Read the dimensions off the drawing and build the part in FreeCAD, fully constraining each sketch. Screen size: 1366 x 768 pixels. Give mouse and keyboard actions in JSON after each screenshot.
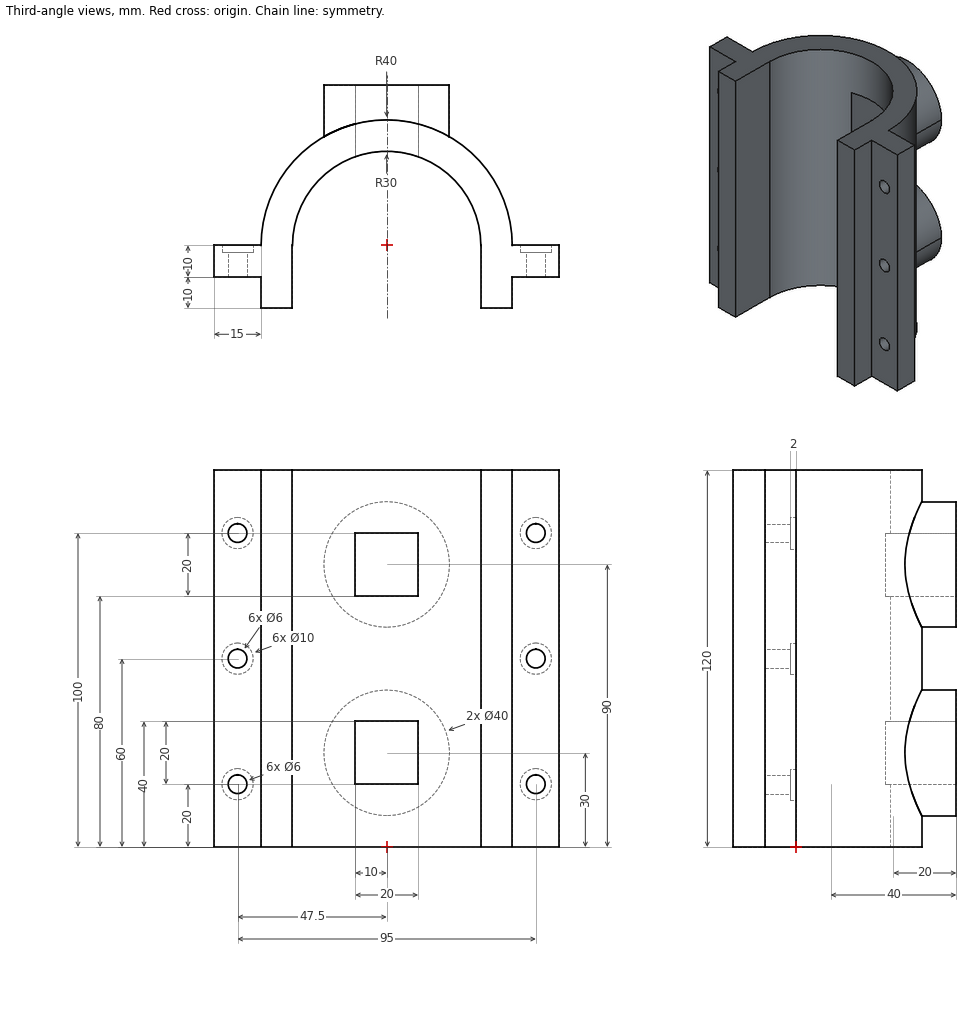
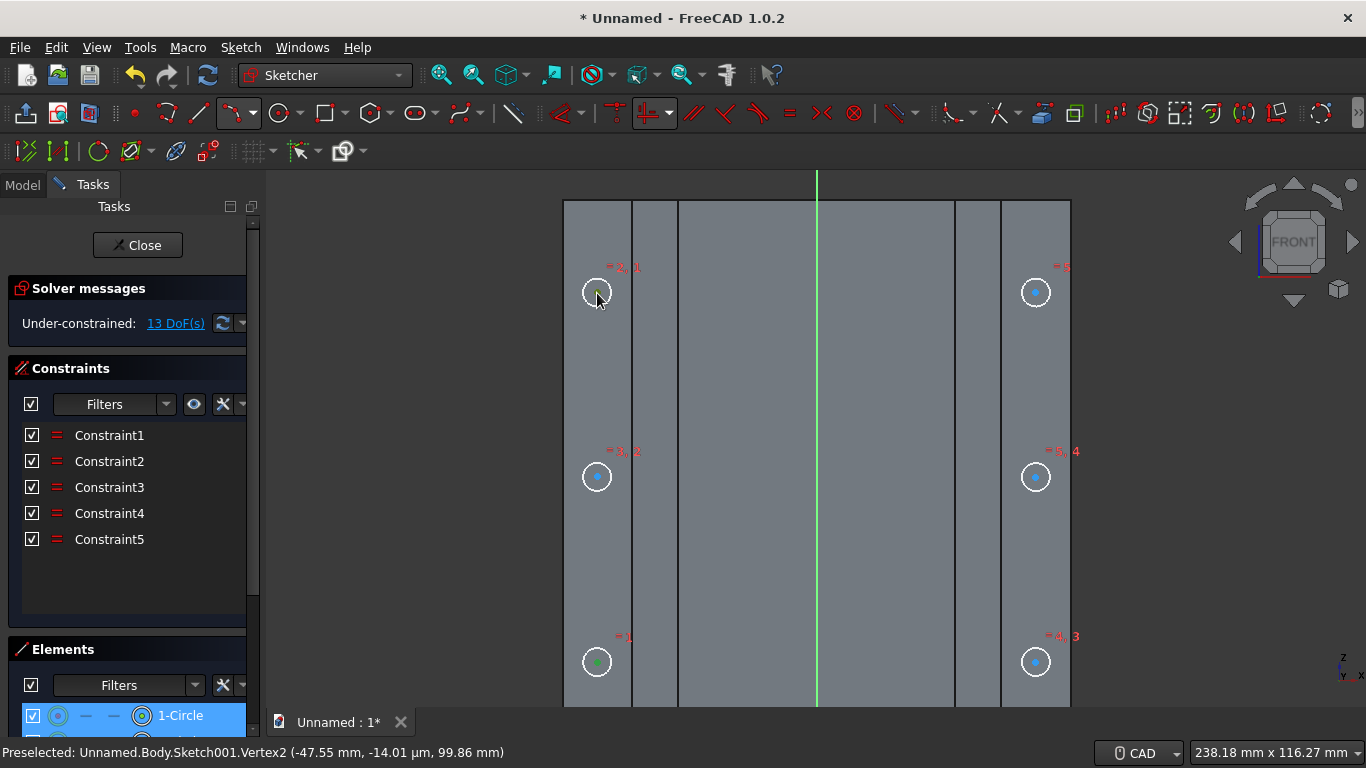
{"action": "left_click", "coordinate": [672, 114]}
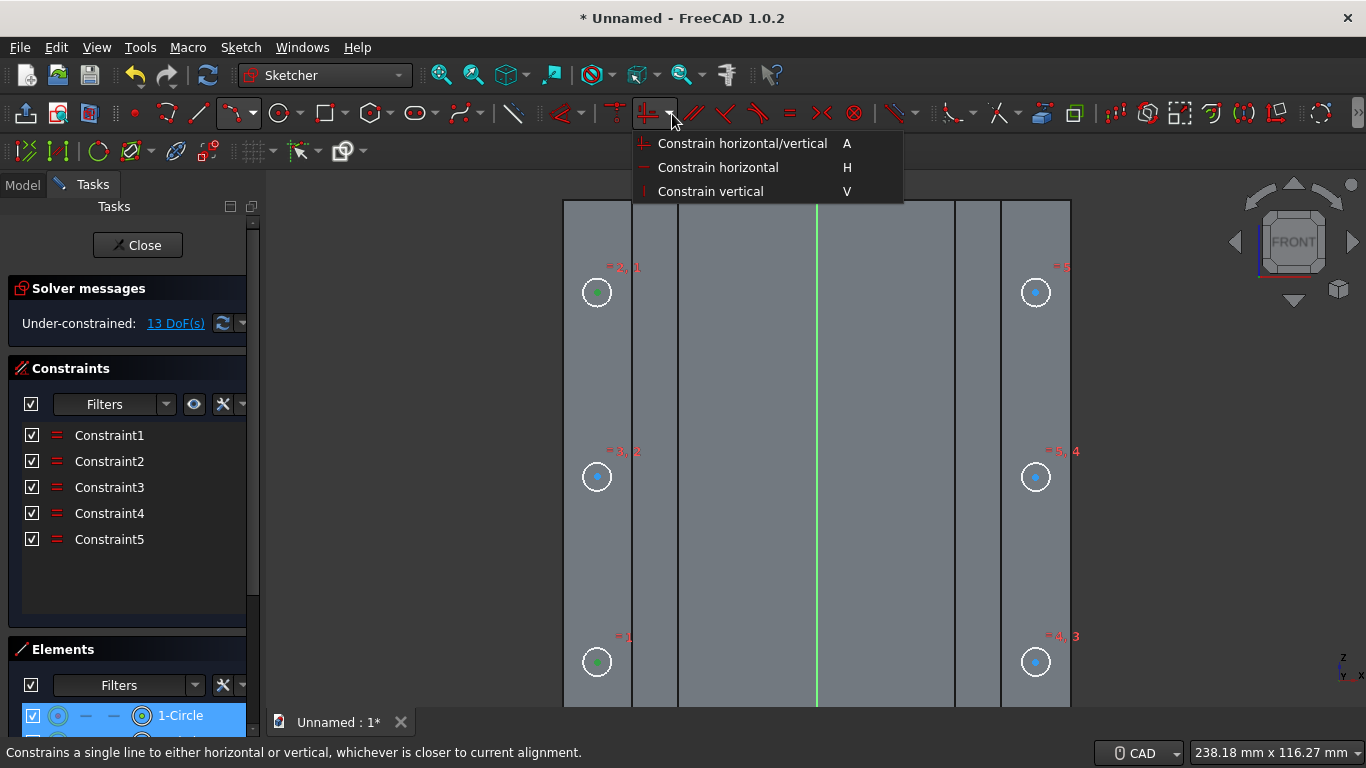
{"action": "left_click", "coordinate": [768, 191]}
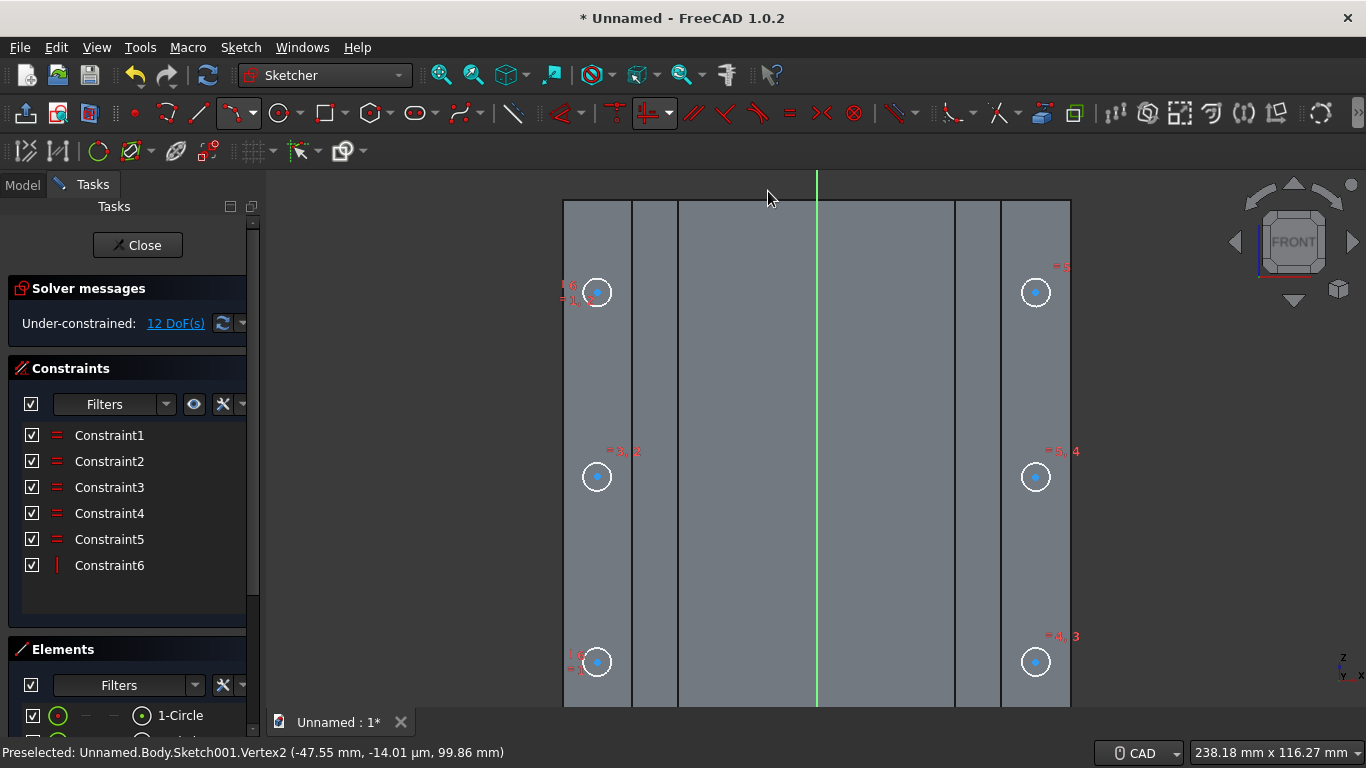
{"action": "left_click", "coordinate": [597, 662]}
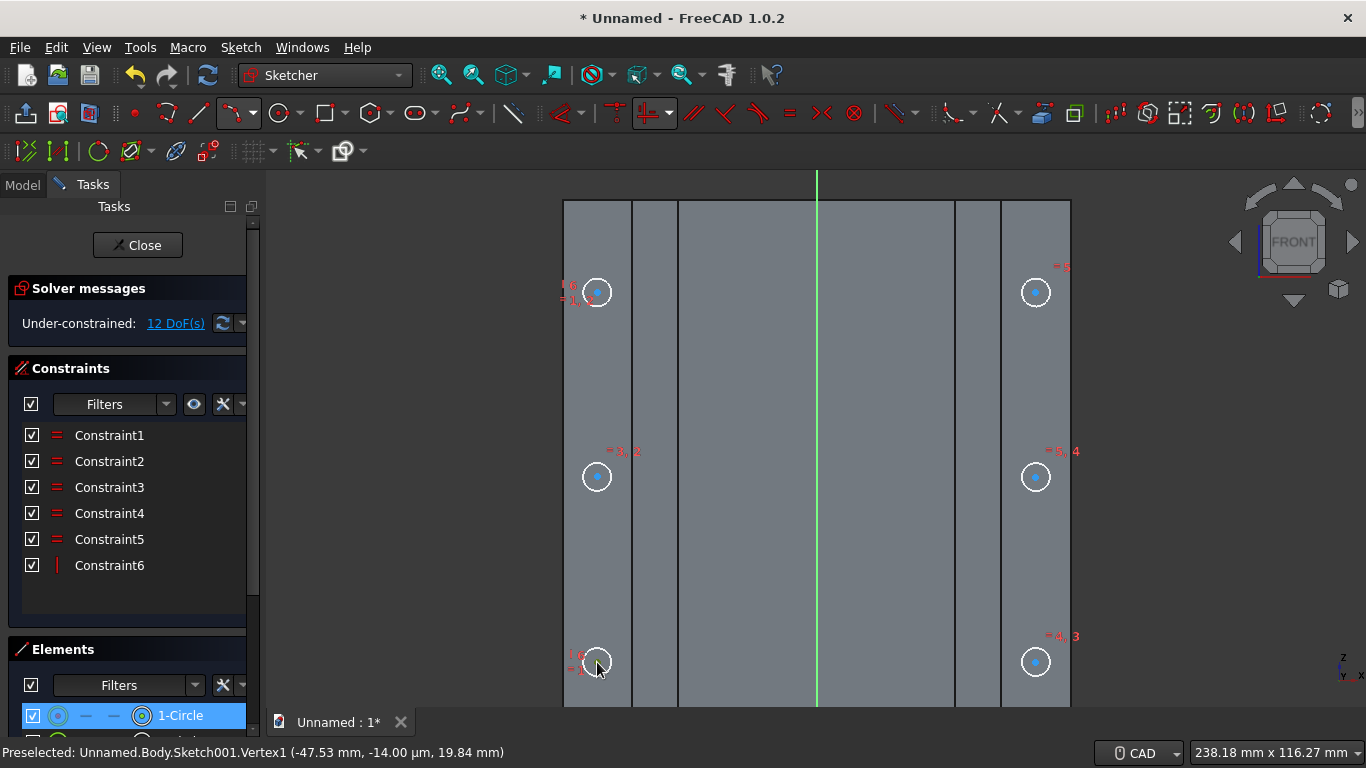
{"action": "left_click", "coordinate": [597, 477]}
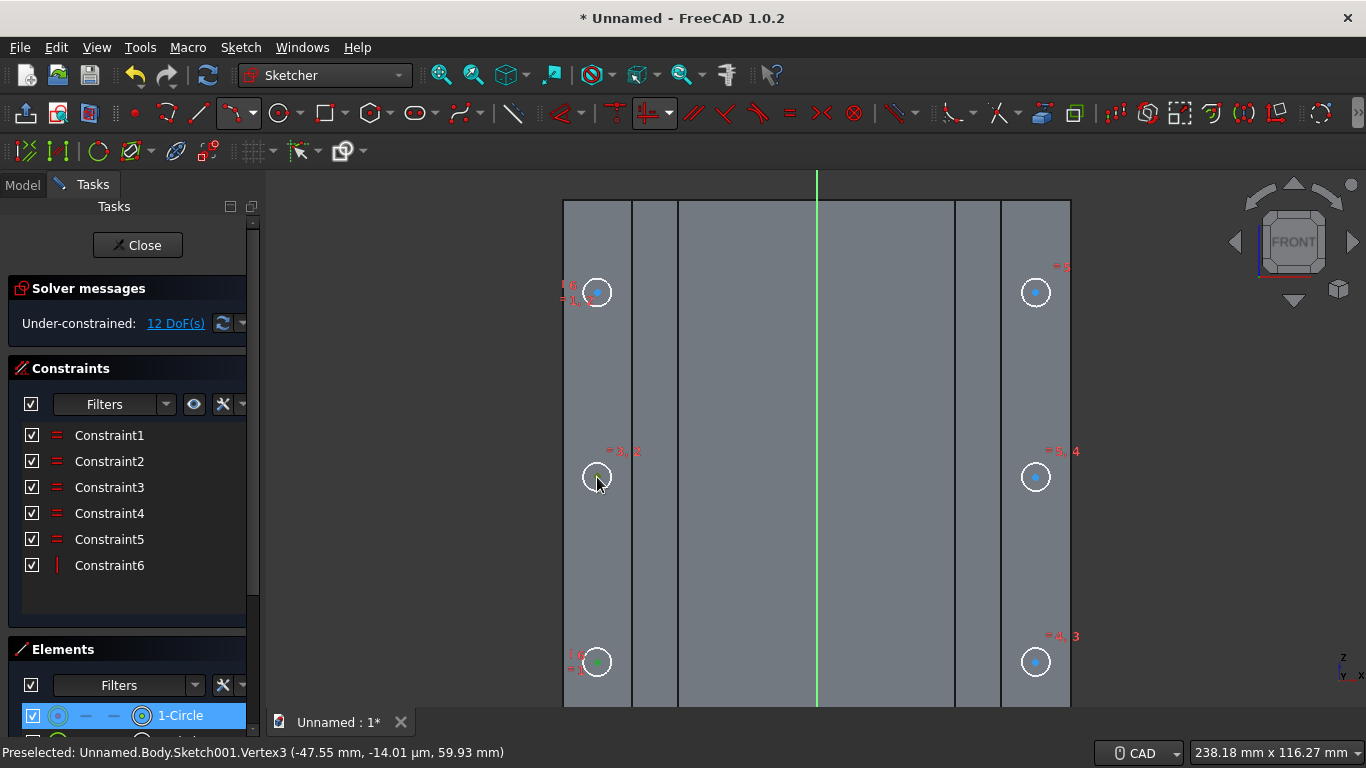
{"action": "left_click", "coordinate": [672, 114]}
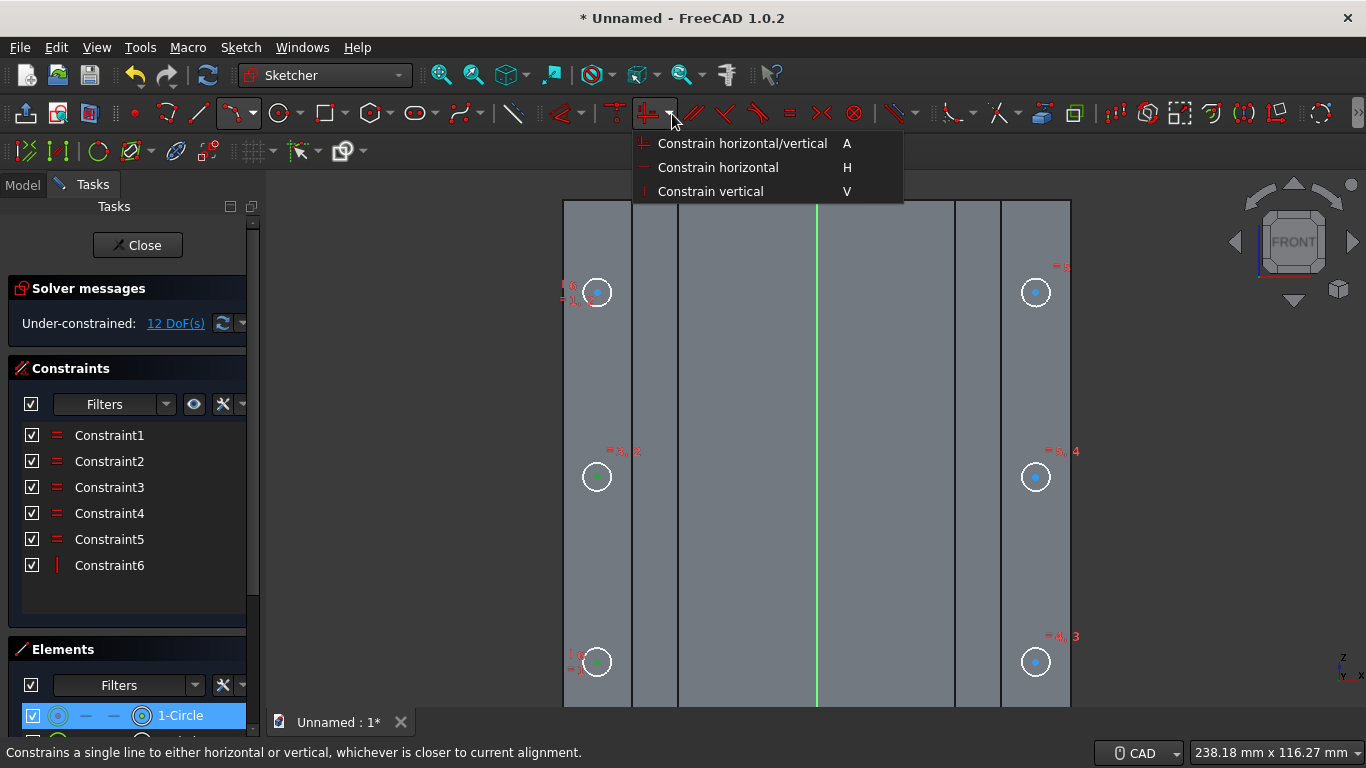
{"action": "left_click", "coordinate": [768, 191]}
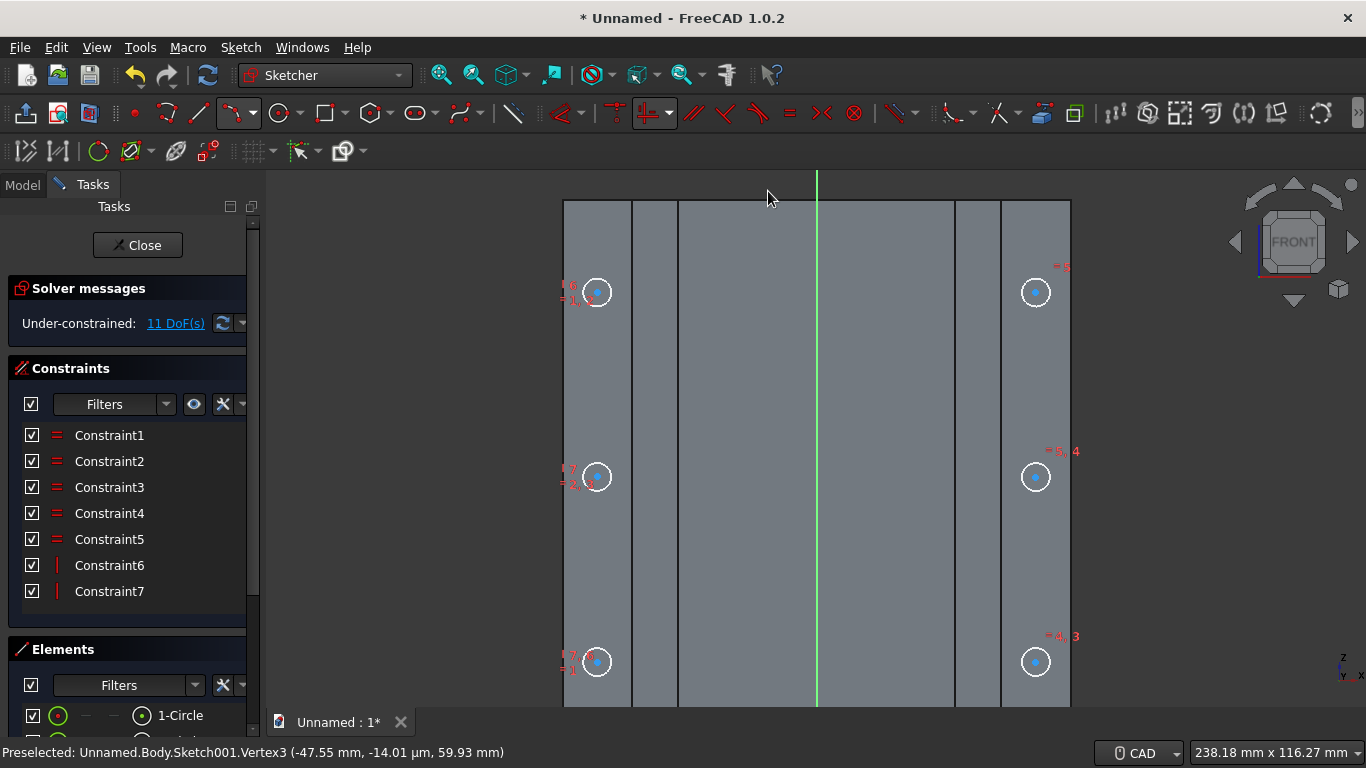
{"action": "left_click", "coordinate": [597, 662]}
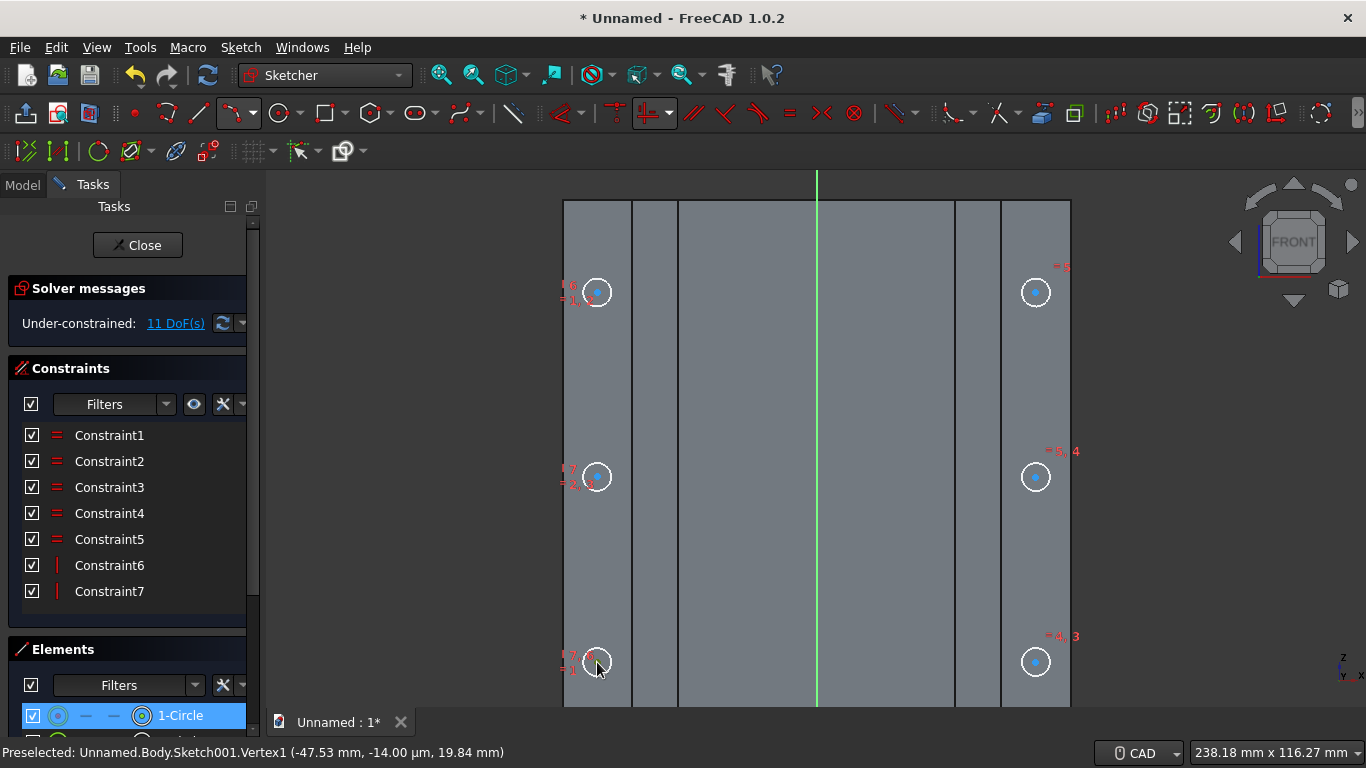
{"action": "left_click", "coordinate": [1036, 662]}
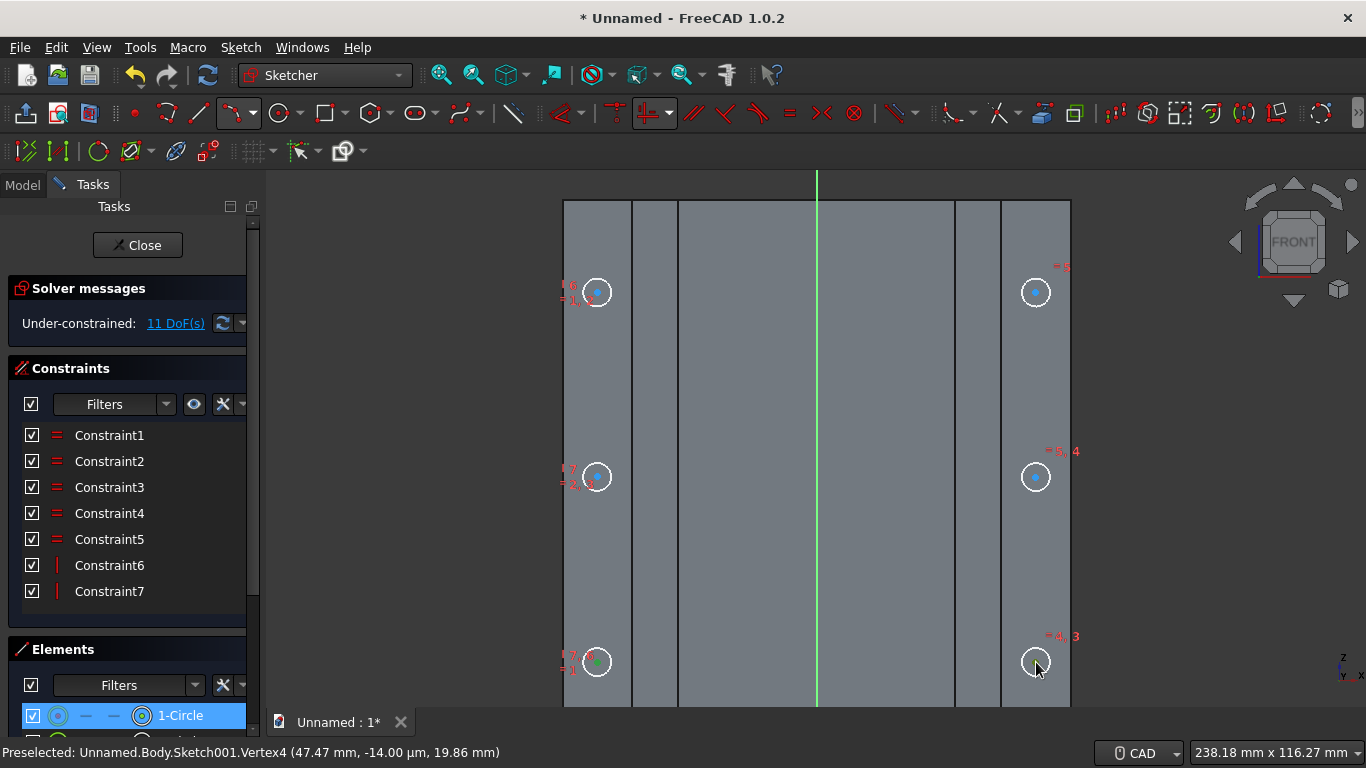
{"action": "key", "text": "h"}